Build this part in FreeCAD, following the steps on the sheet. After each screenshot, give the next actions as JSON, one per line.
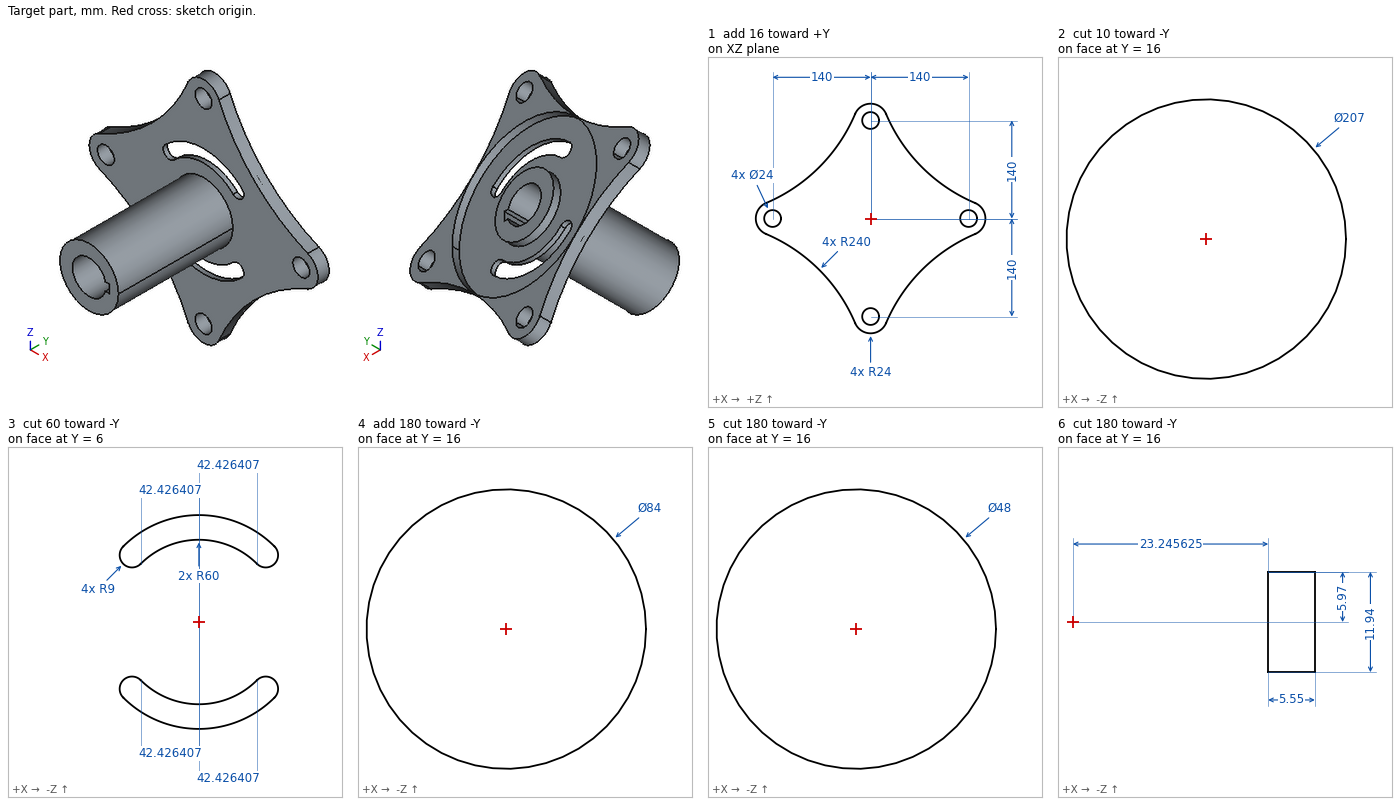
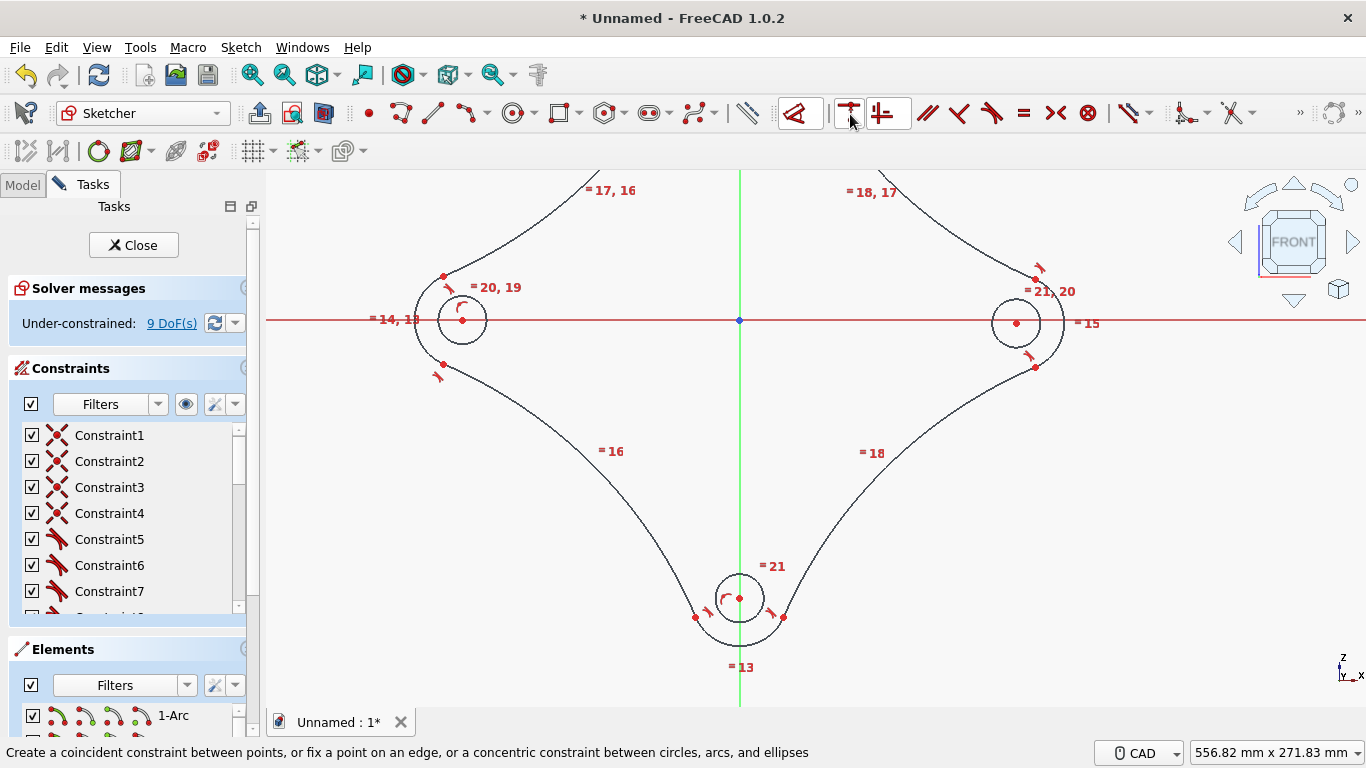
{"action": "scroll", "coordinate": [757, 582], "scroll_direction": "down", "scroll_amount": 3}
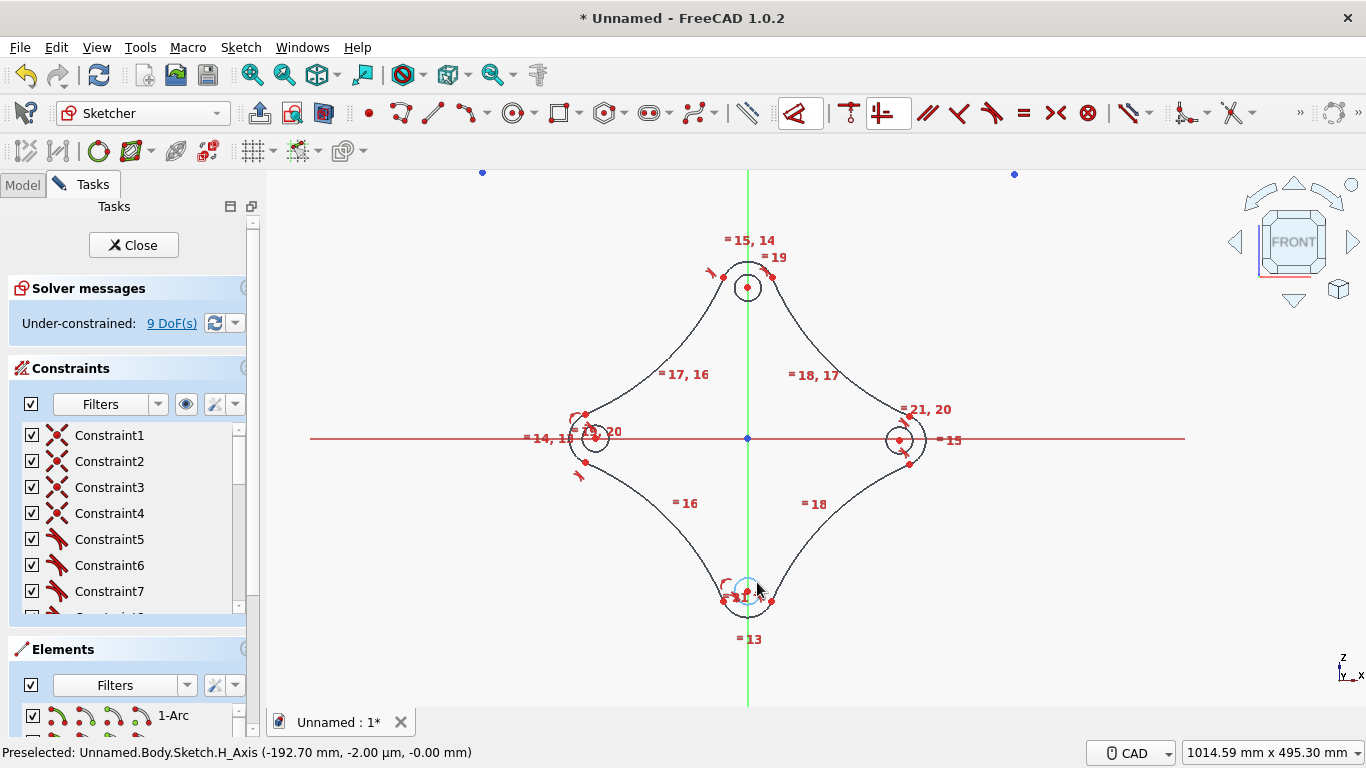
{"action": "left_click", "coordinate": [748, 288]}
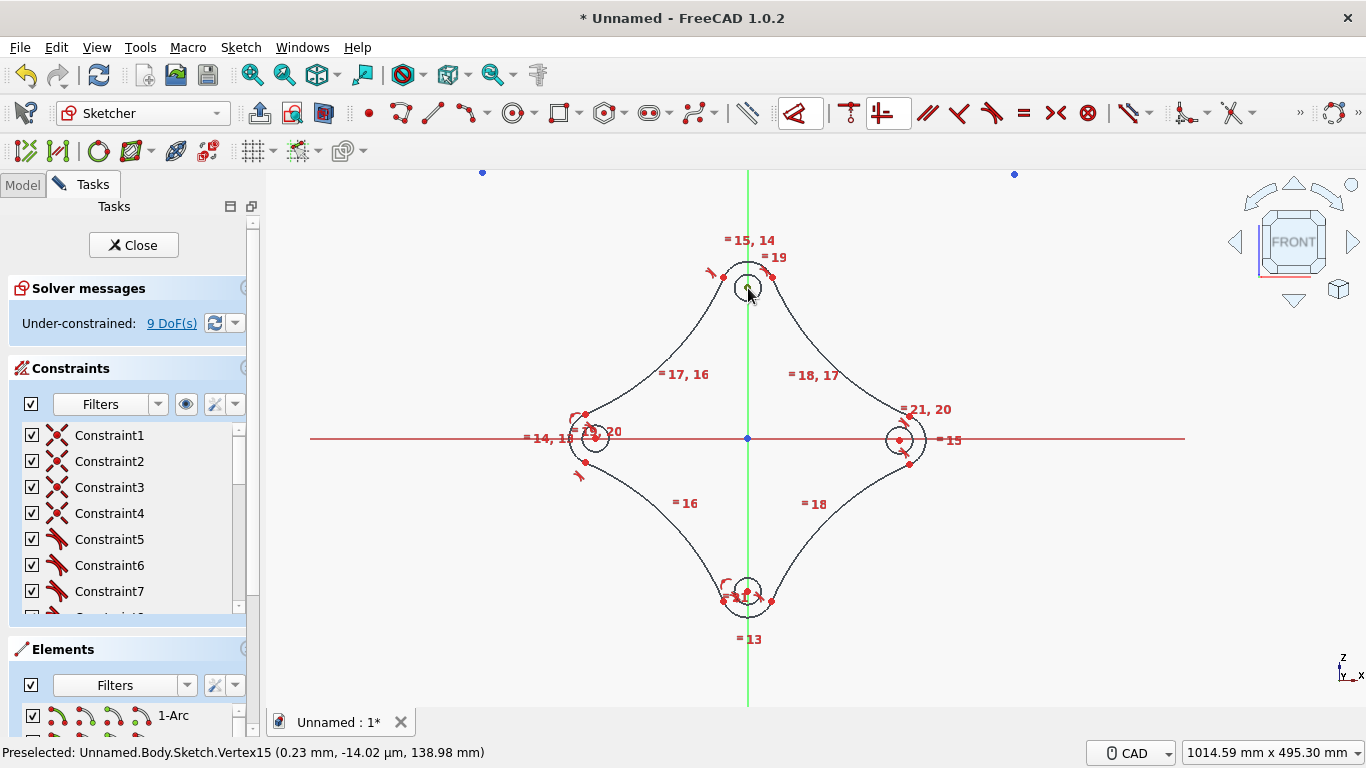
{"action": "left_click", "coordinate": [748, 542]}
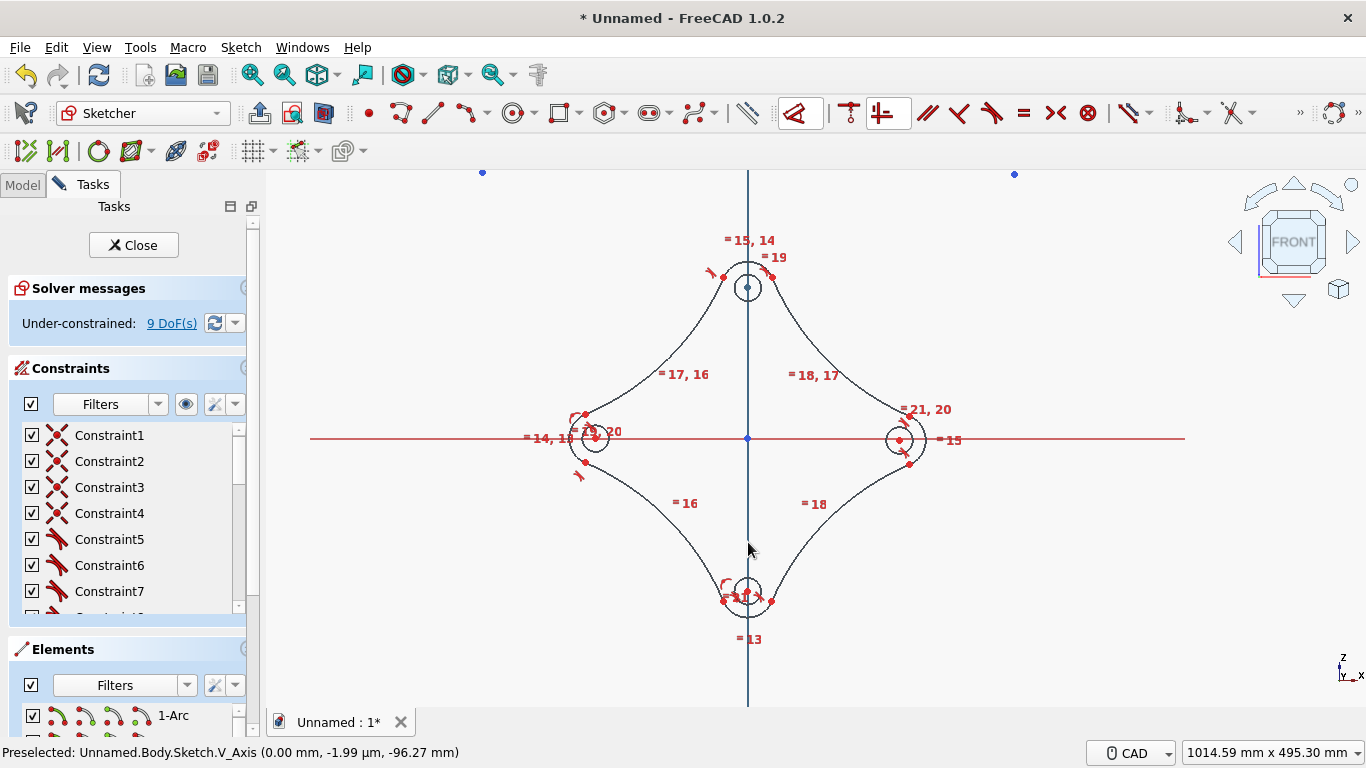
{"action": "left_click", "coordinate": [850, 114]}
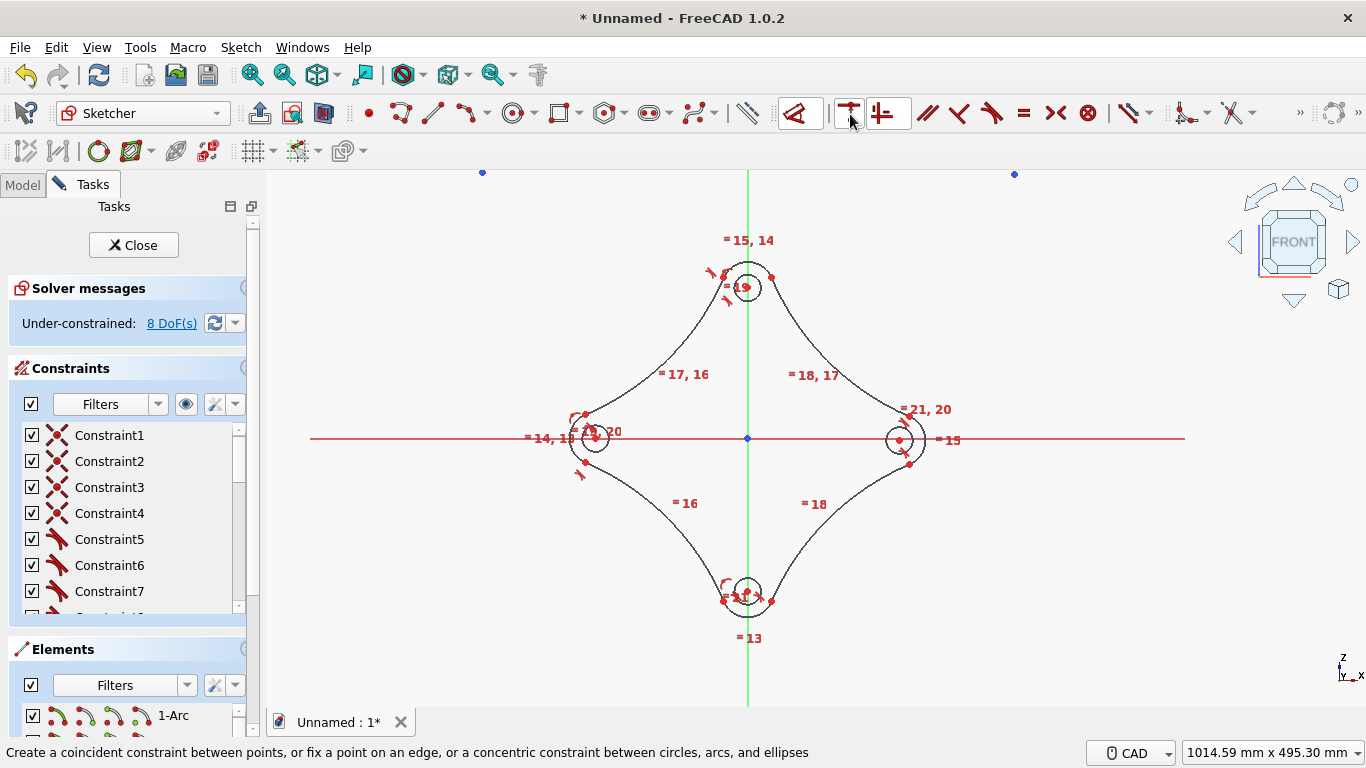
{"action": "left_click", "coordinate": [900, 441]}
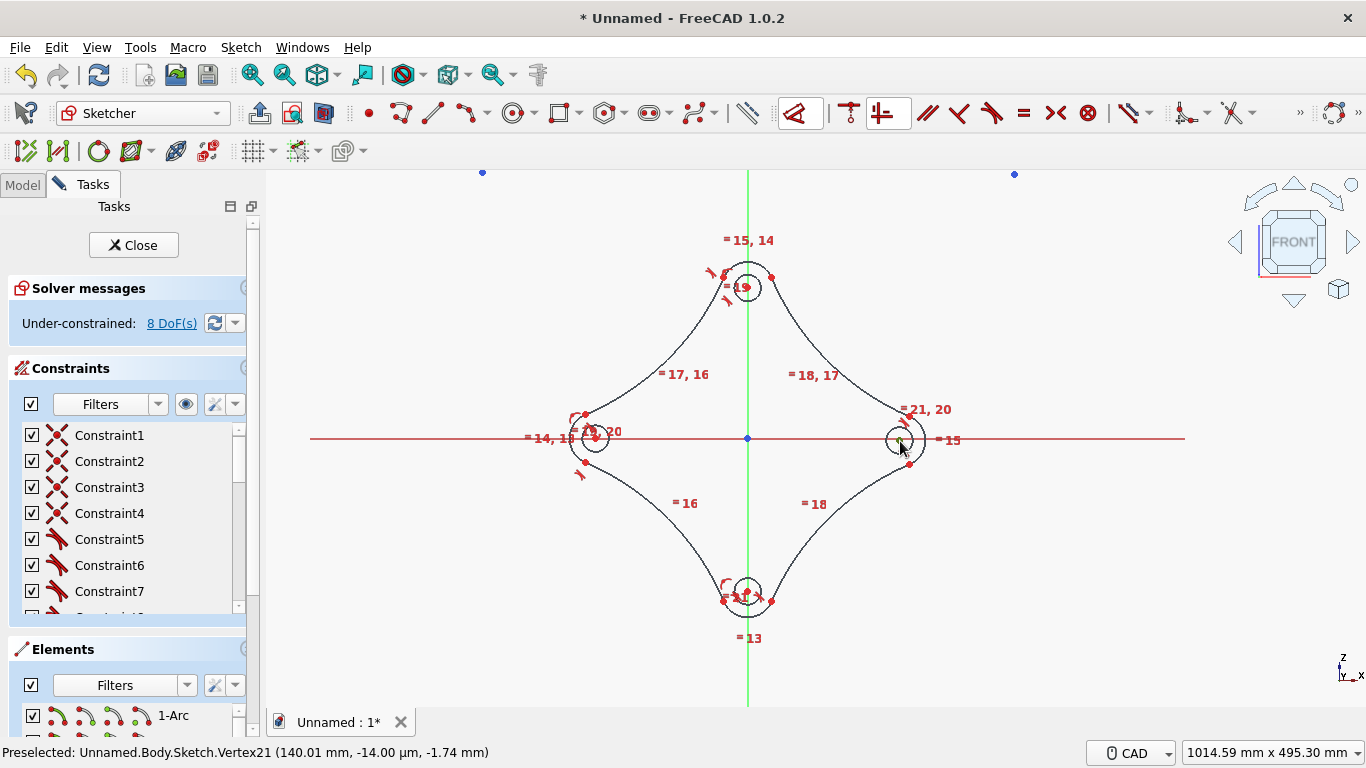
{"action": "left_click", "coordinate": [359, 439]}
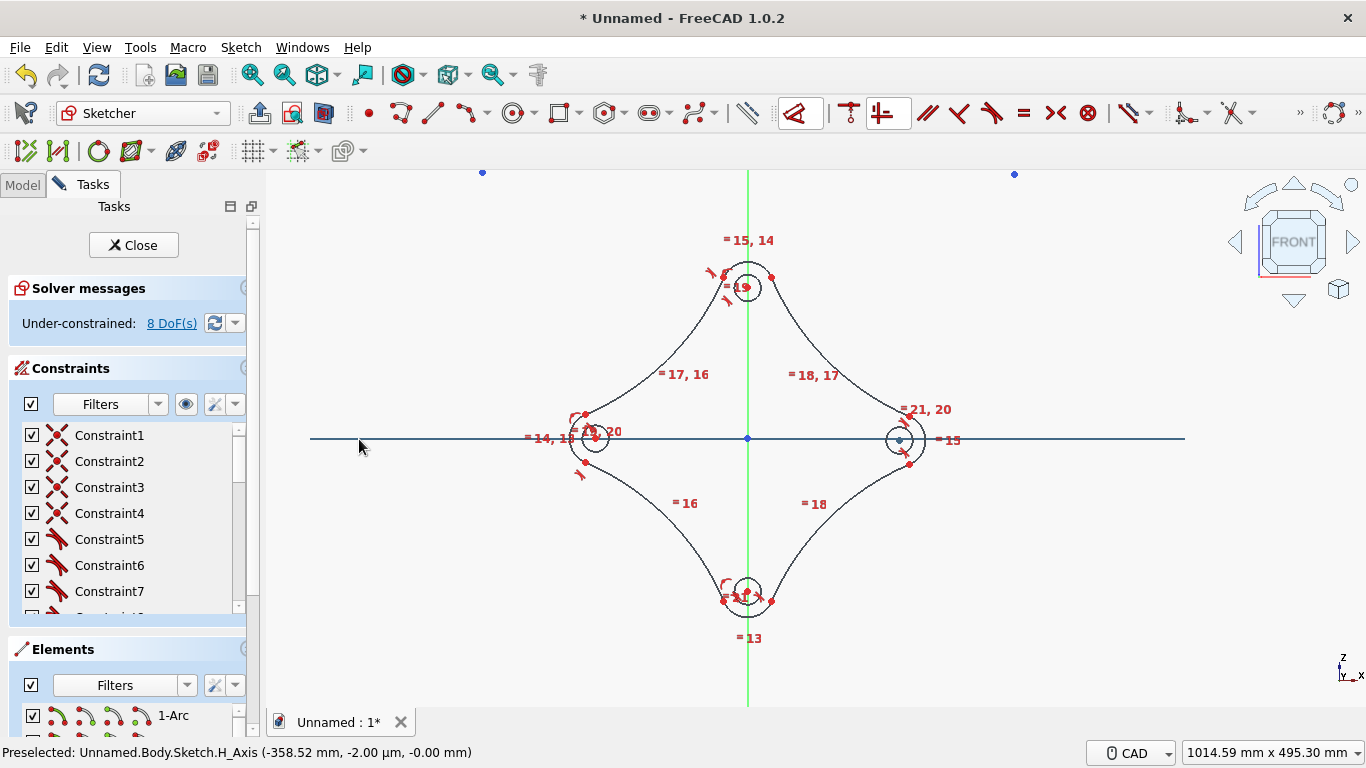
{"action": "left_click", "coordinate": [850, 114]}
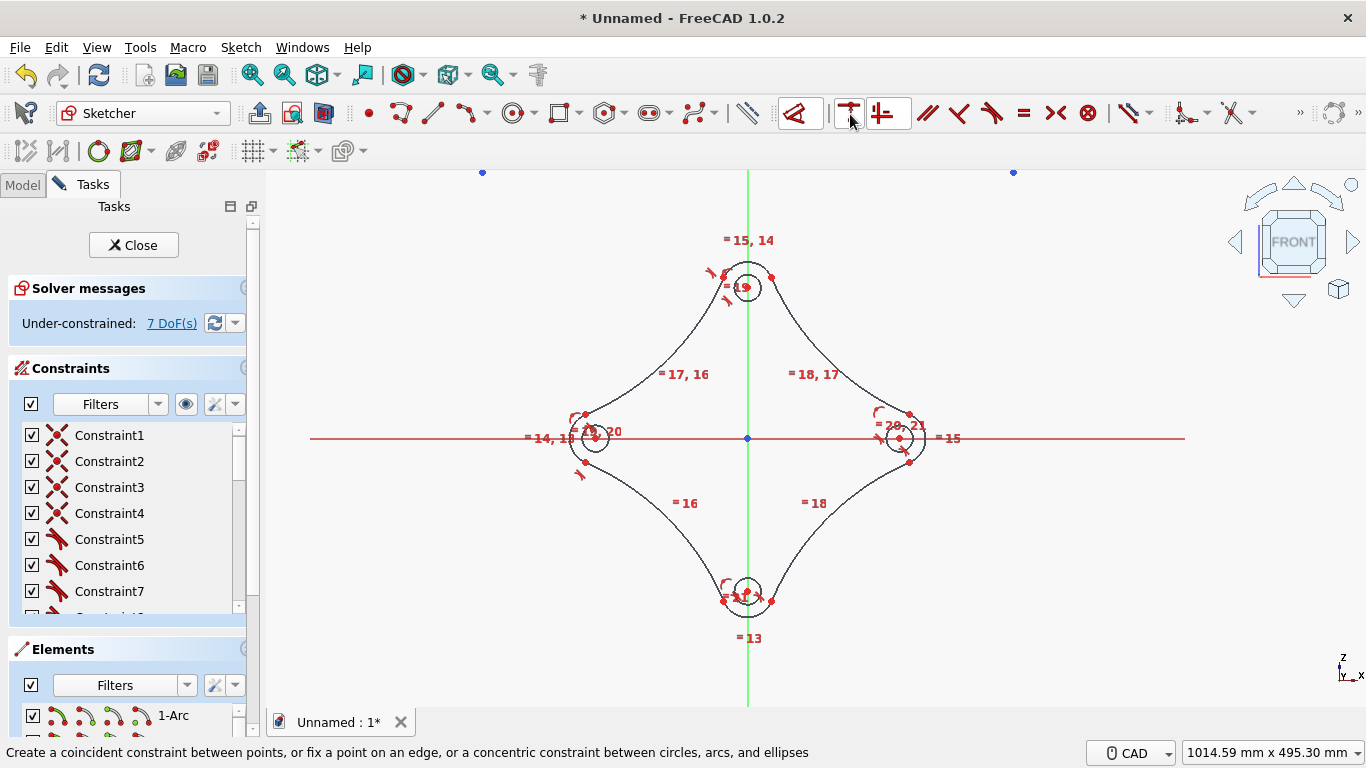
{"action": "scroll", "coordinate": [736, 615], "scroll_direction": "up", "scroll_amount": 3}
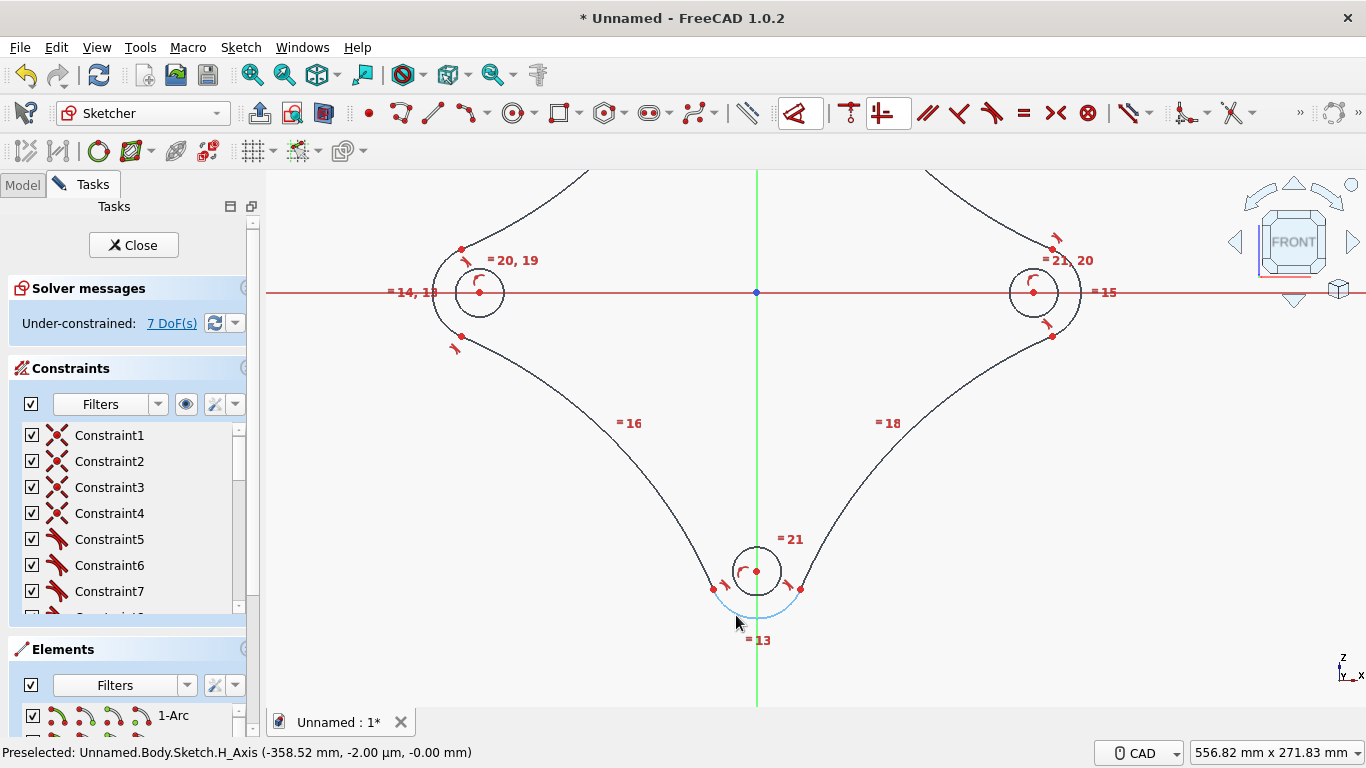
{"action": "left_click", "coordinate": [736, 613]}